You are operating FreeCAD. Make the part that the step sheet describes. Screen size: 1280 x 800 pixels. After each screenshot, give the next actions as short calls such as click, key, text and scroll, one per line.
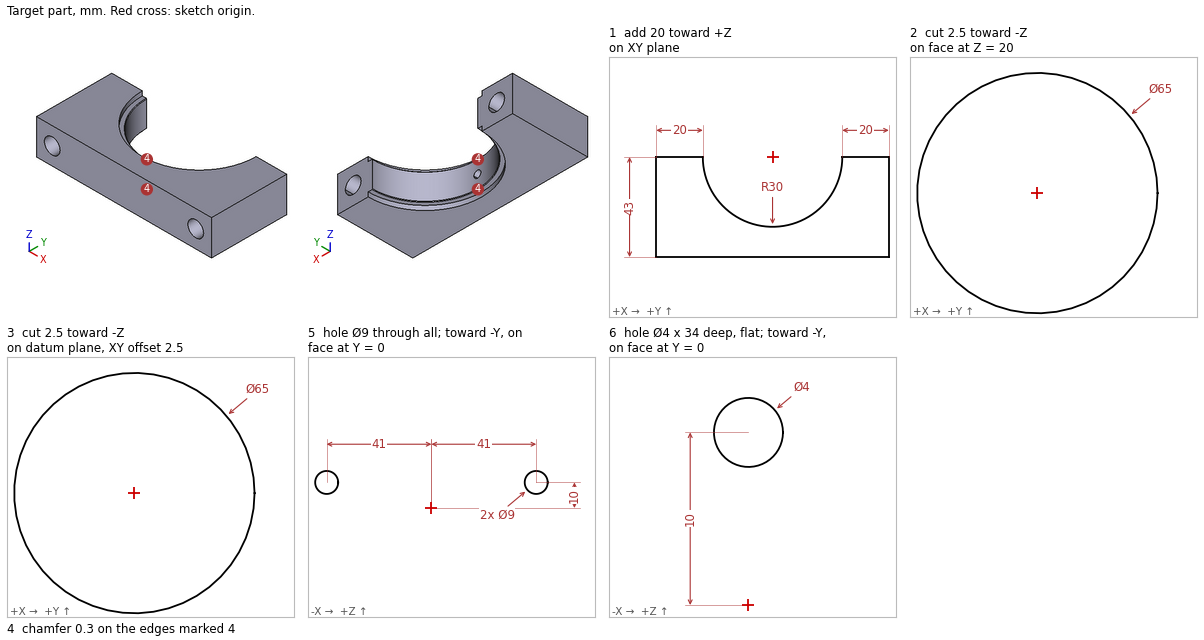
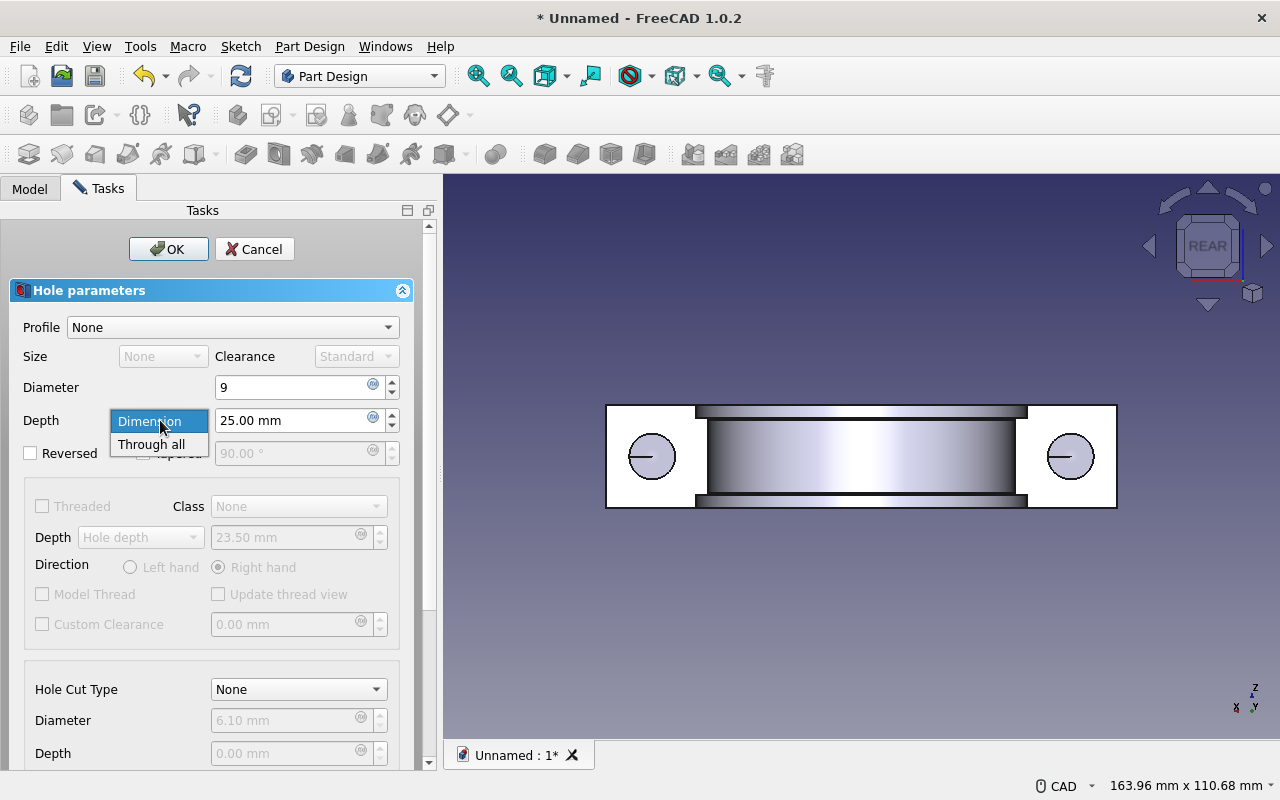
click(158, 444)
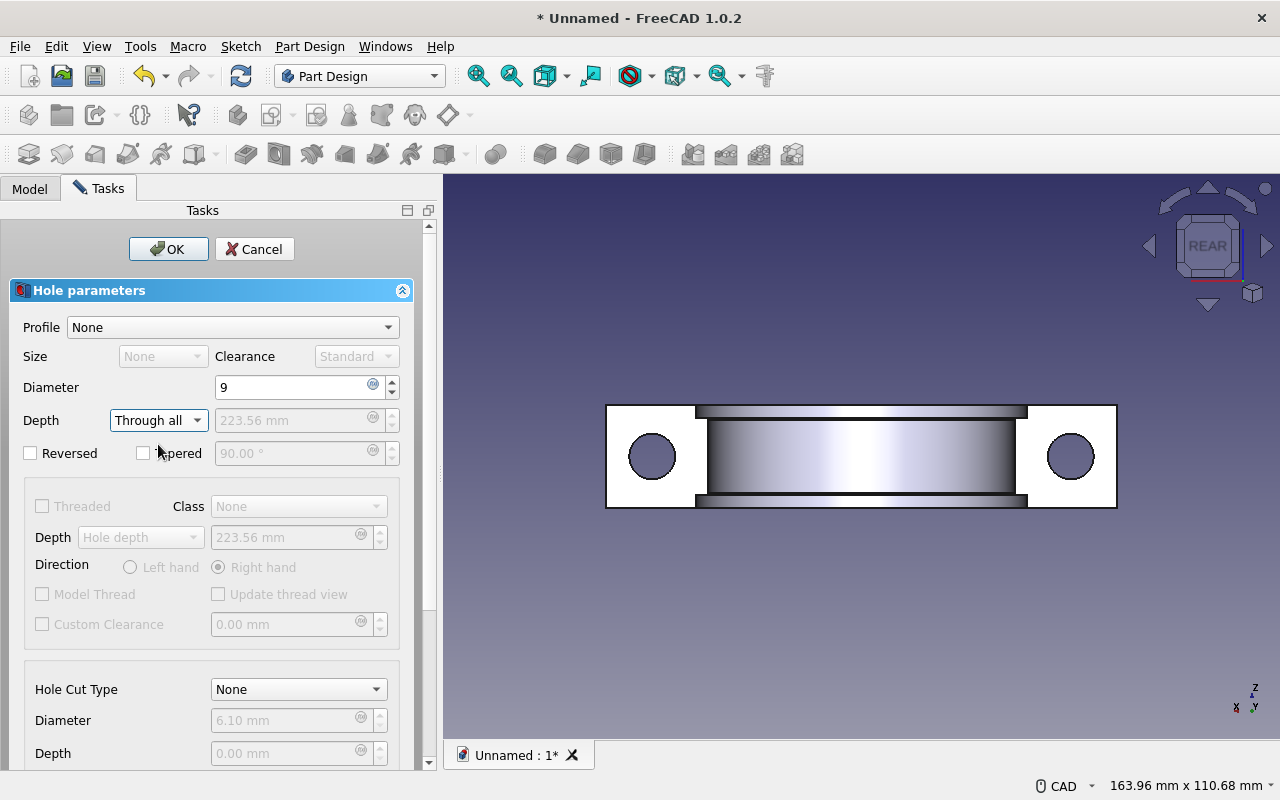
click(169, 249)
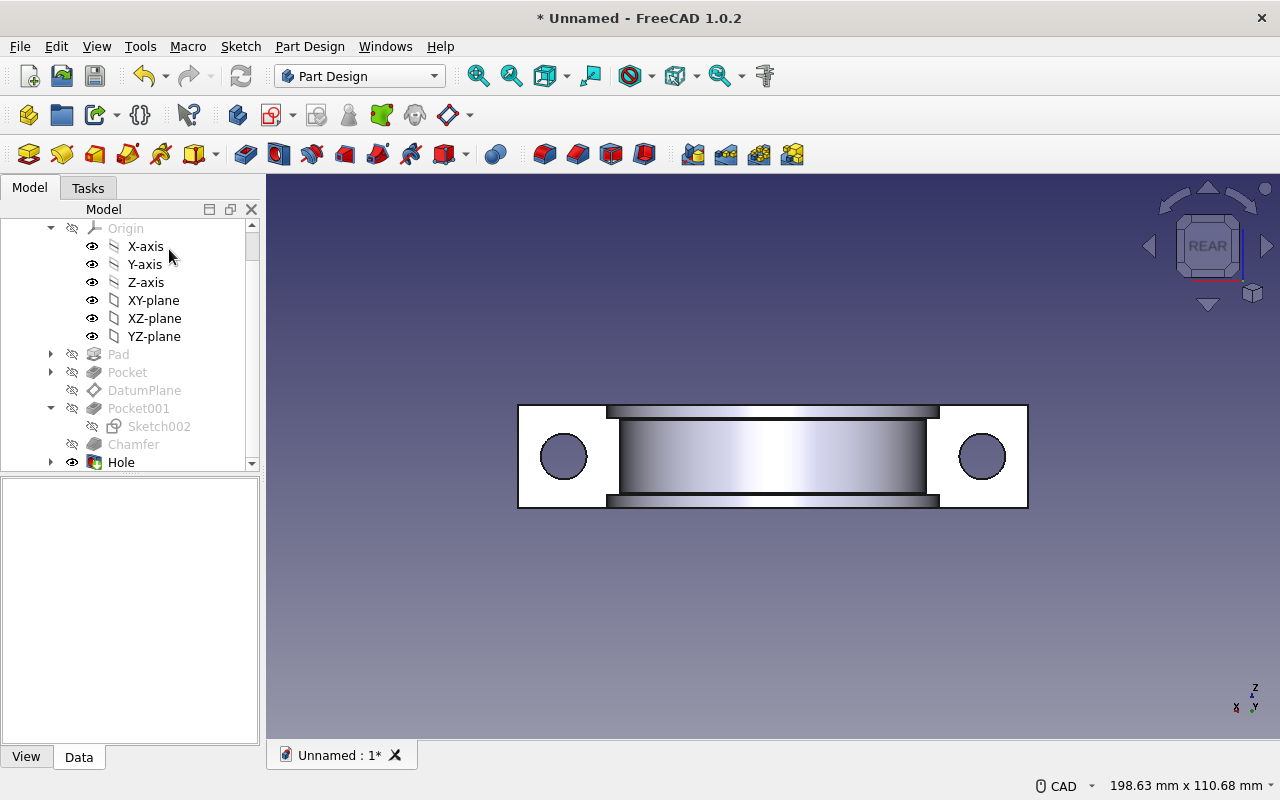
click(540, 426)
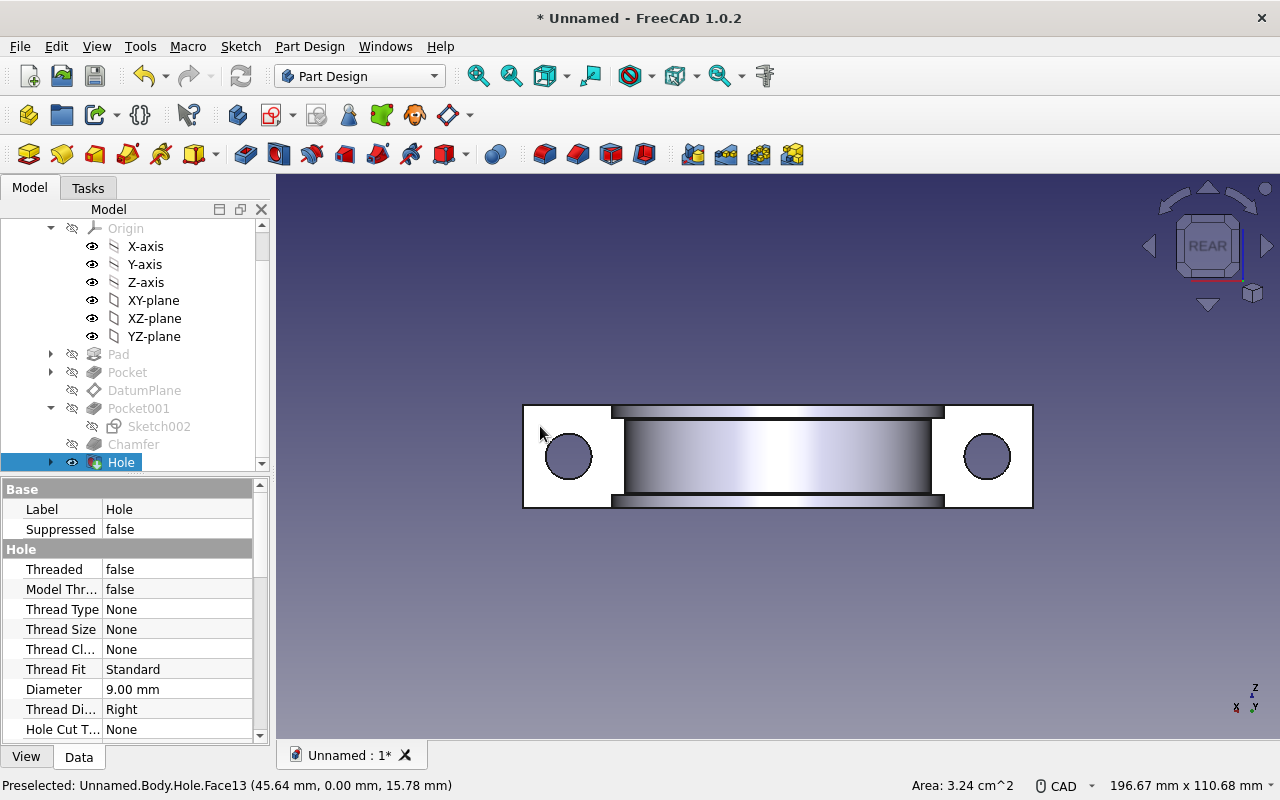
click(270, 116)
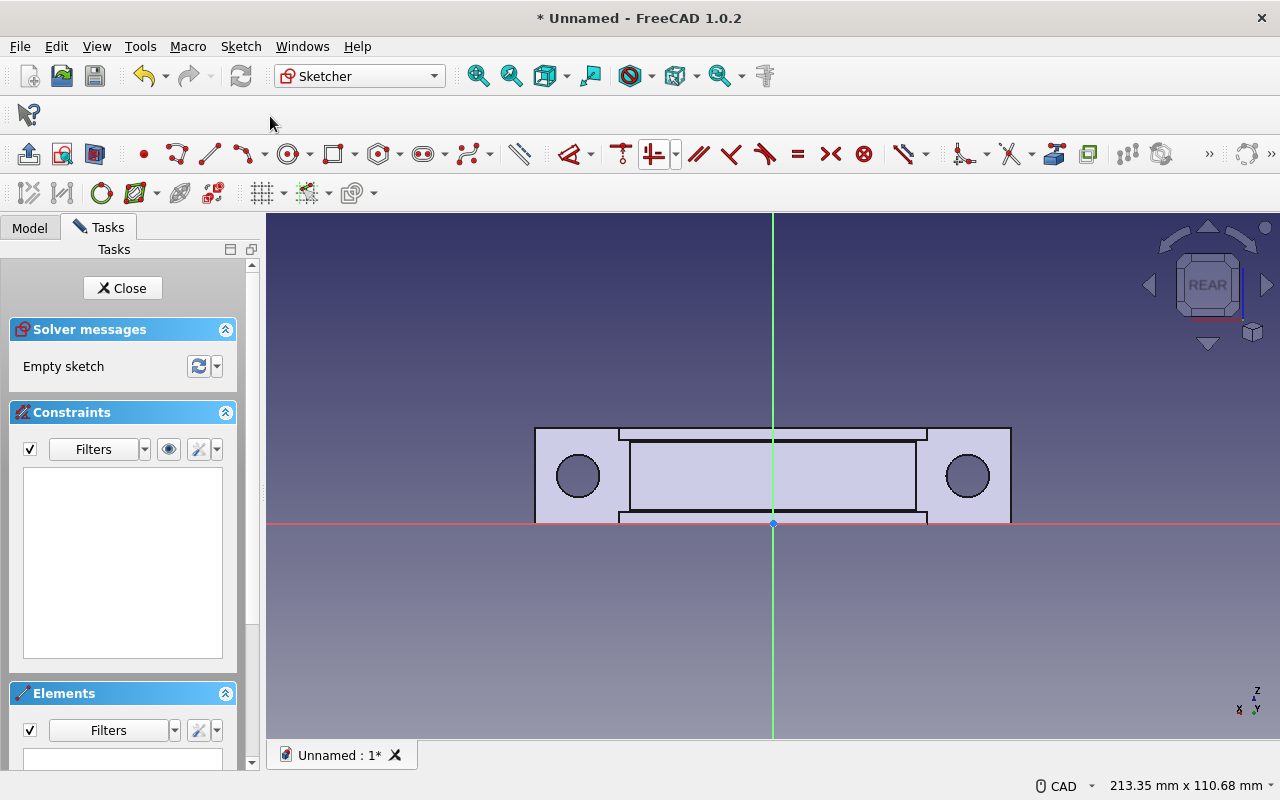
scroll(777, 476, up, 14)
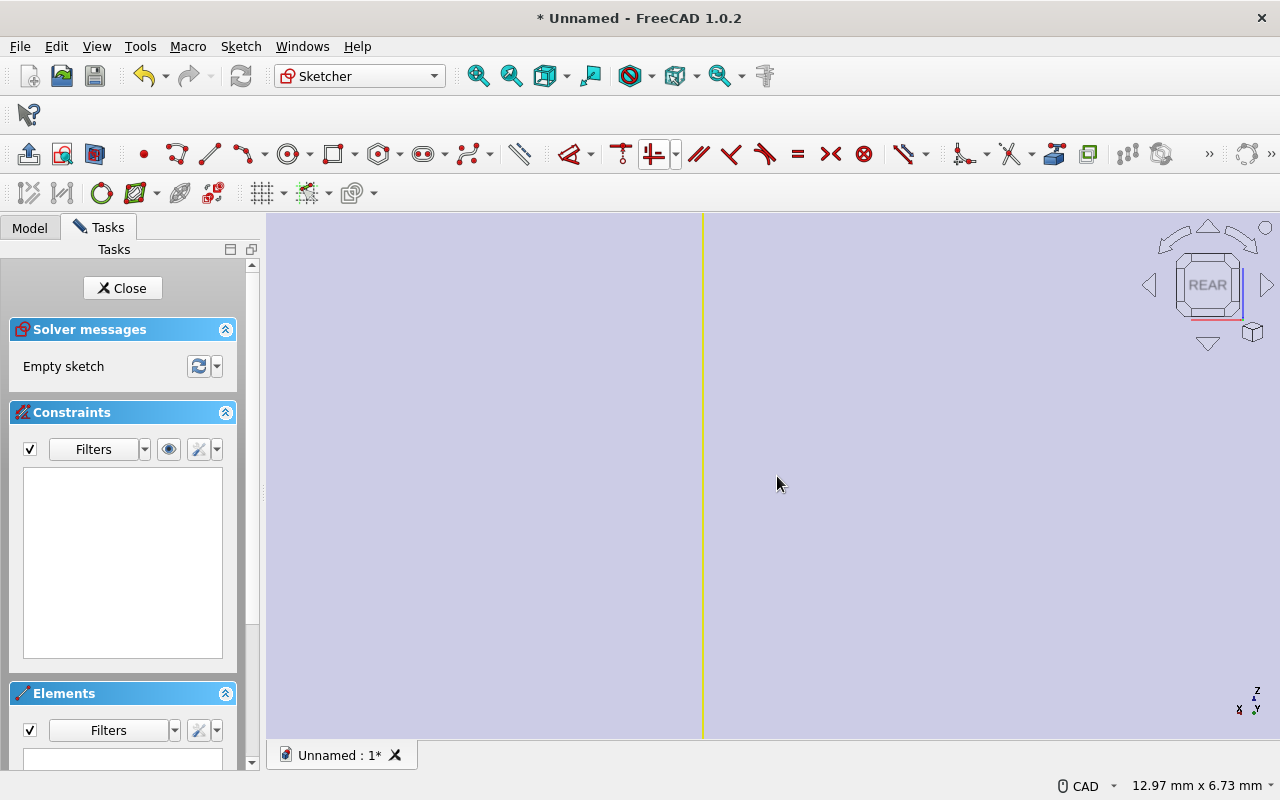
click(288, 154)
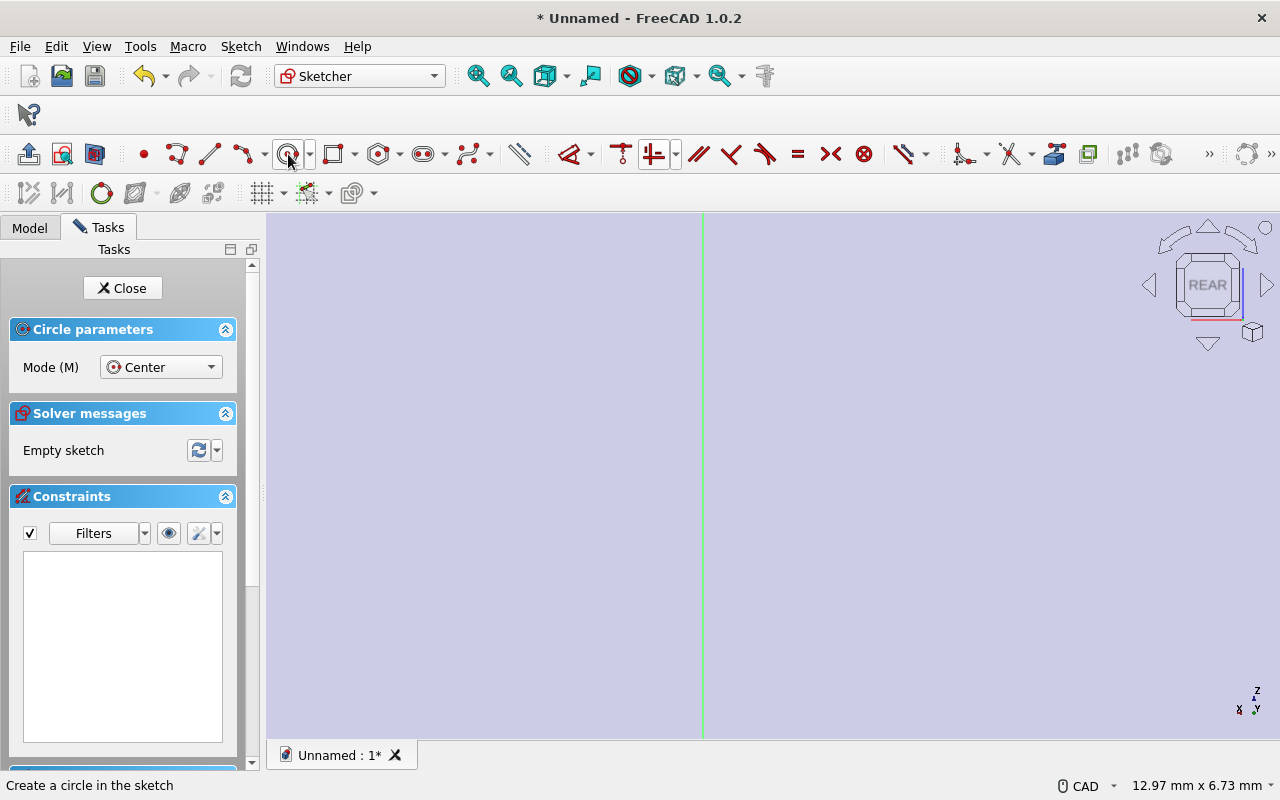
click(703, 468)
click(814, 358)
key(Escape)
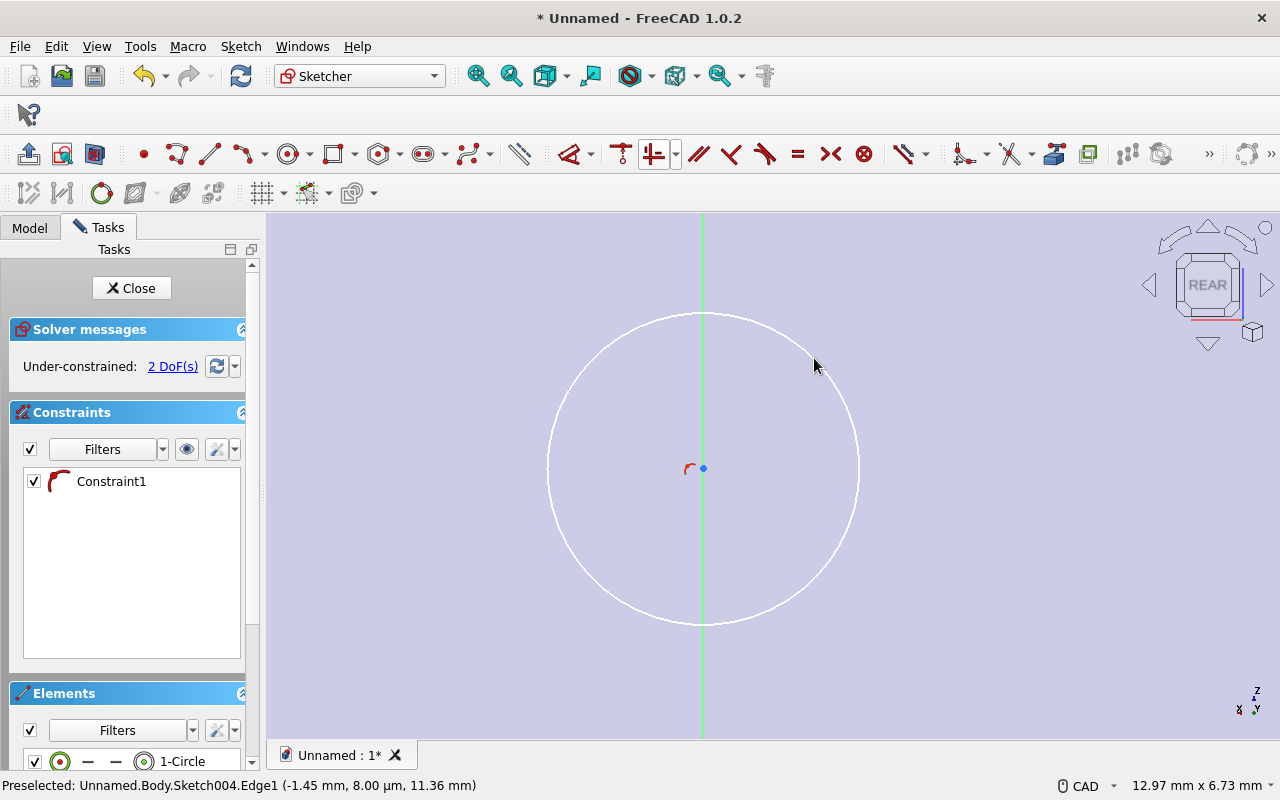
key(d)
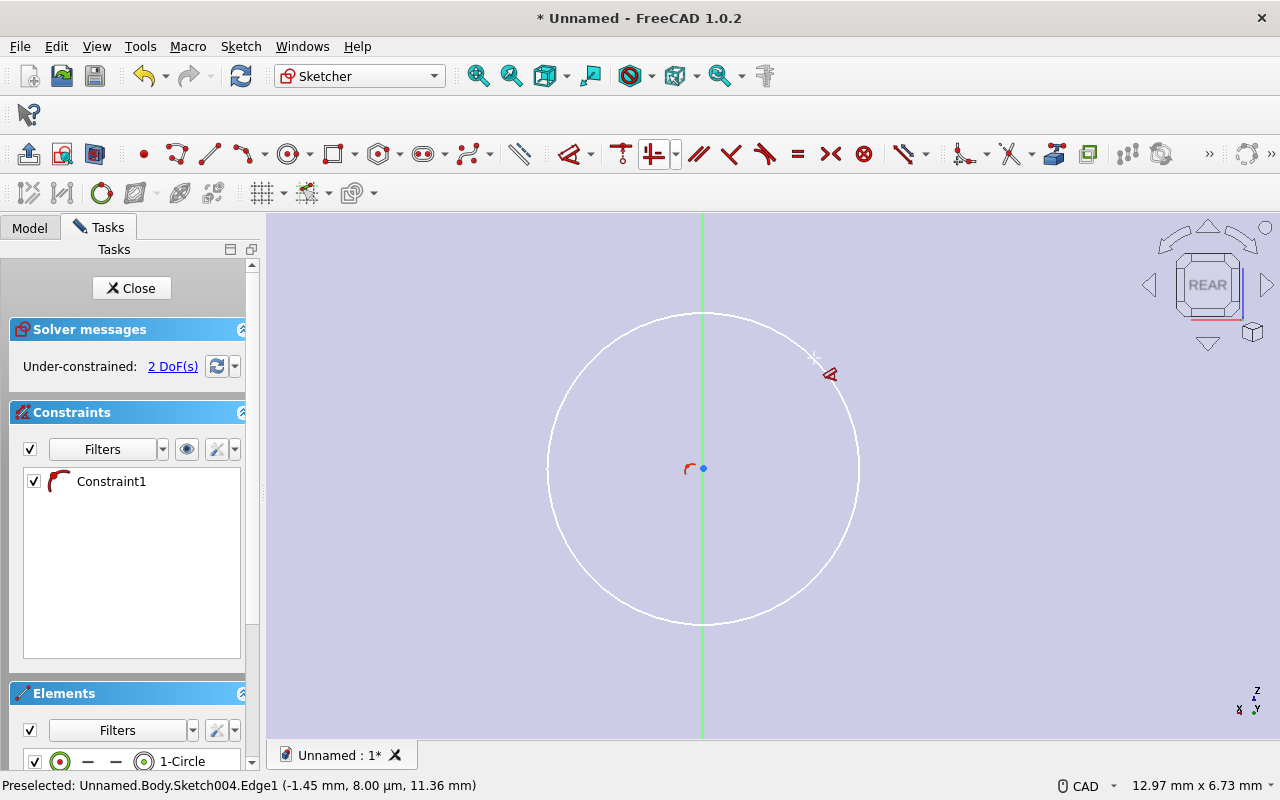
click(813, 358)
click(835, 335)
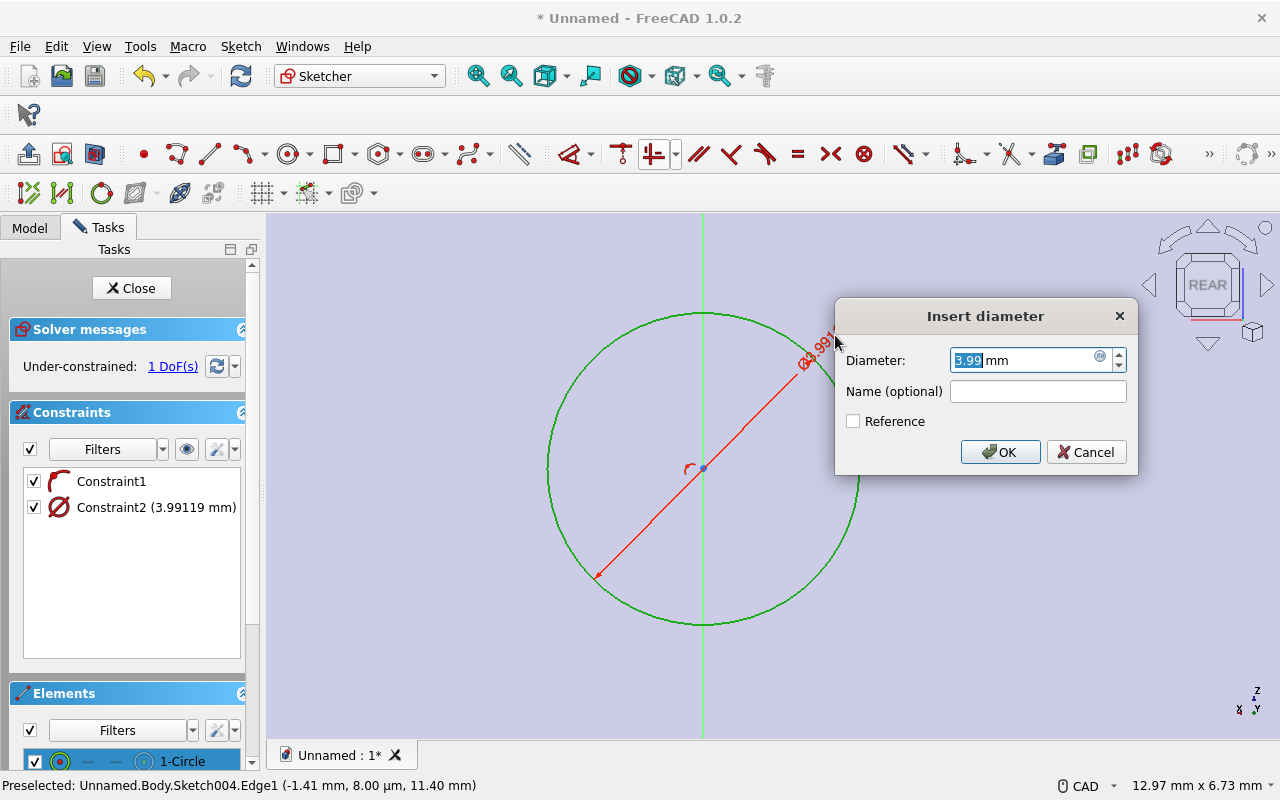
text(4)
key(Return)